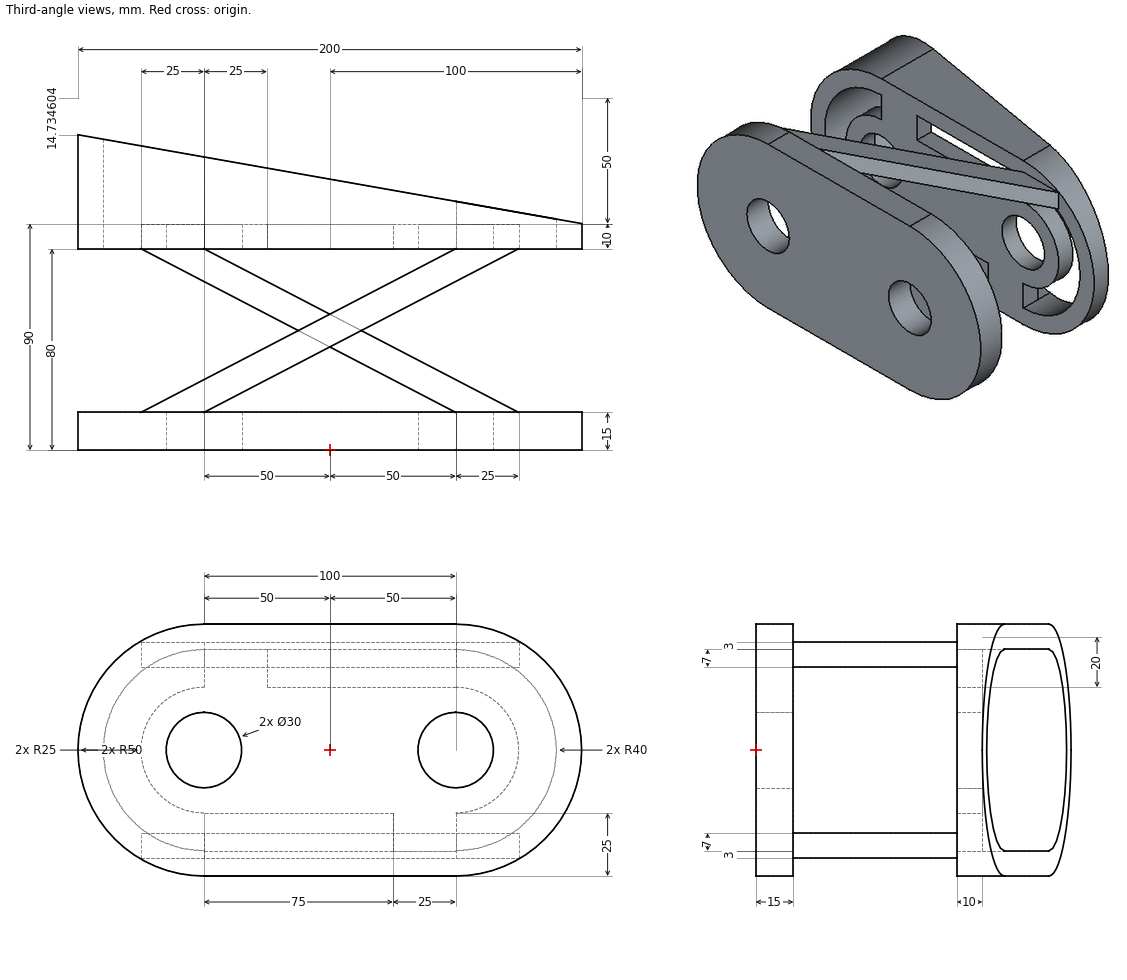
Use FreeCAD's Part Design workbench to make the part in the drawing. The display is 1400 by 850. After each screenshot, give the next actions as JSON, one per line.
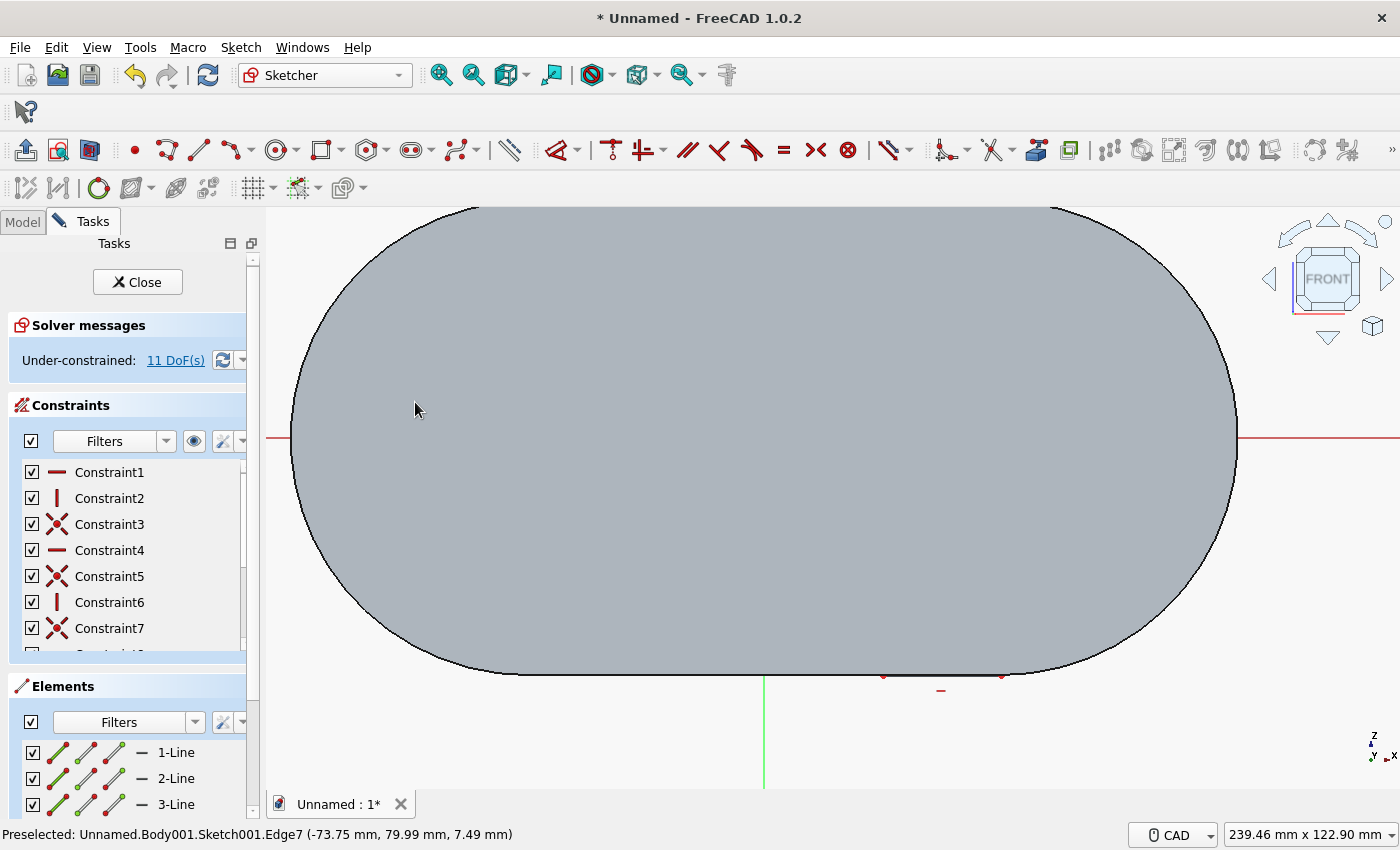
{"action": "left_click", "coordinate": [670, 321]}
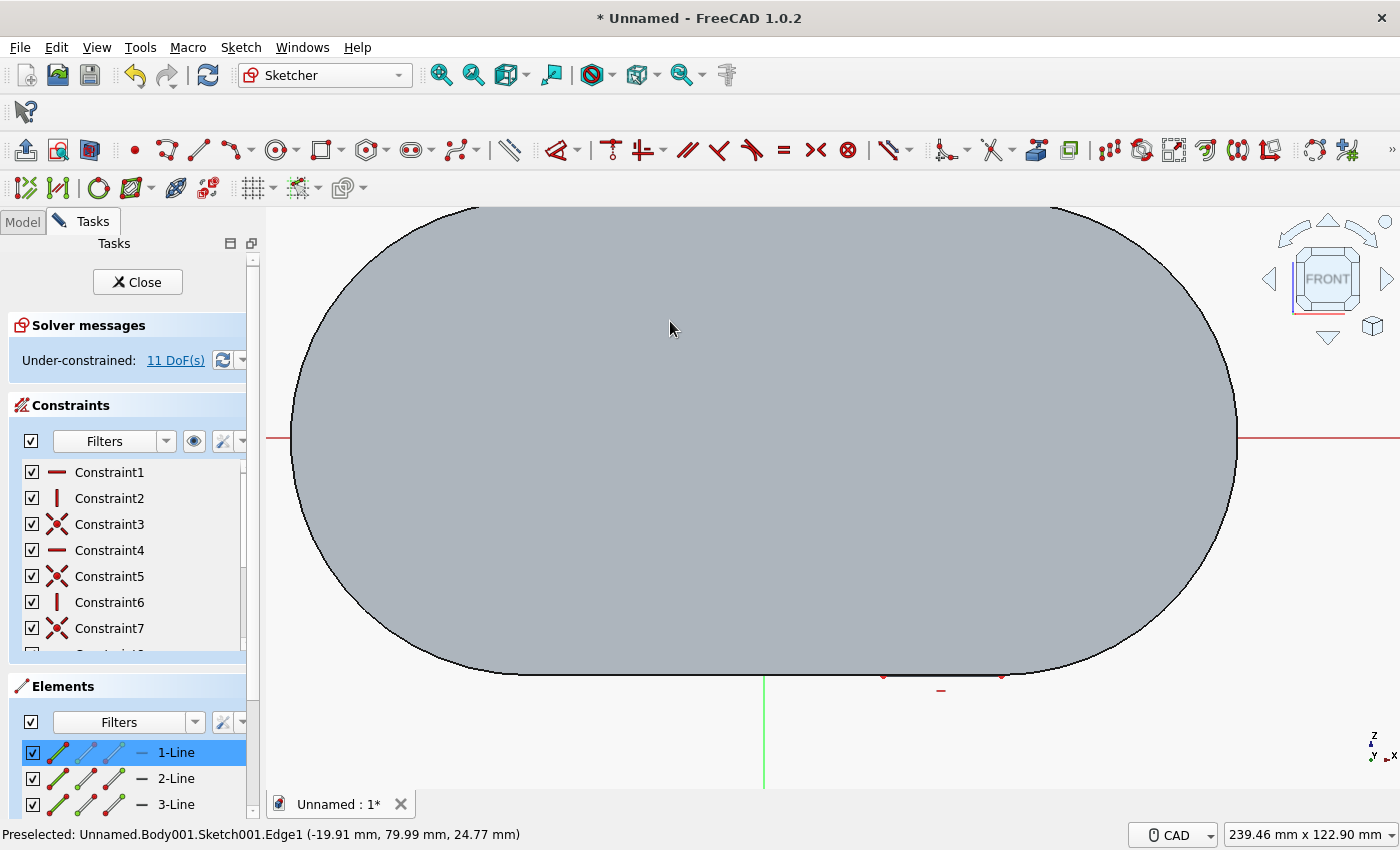
{"action": "left_click", "coordinate": [1097, 509]}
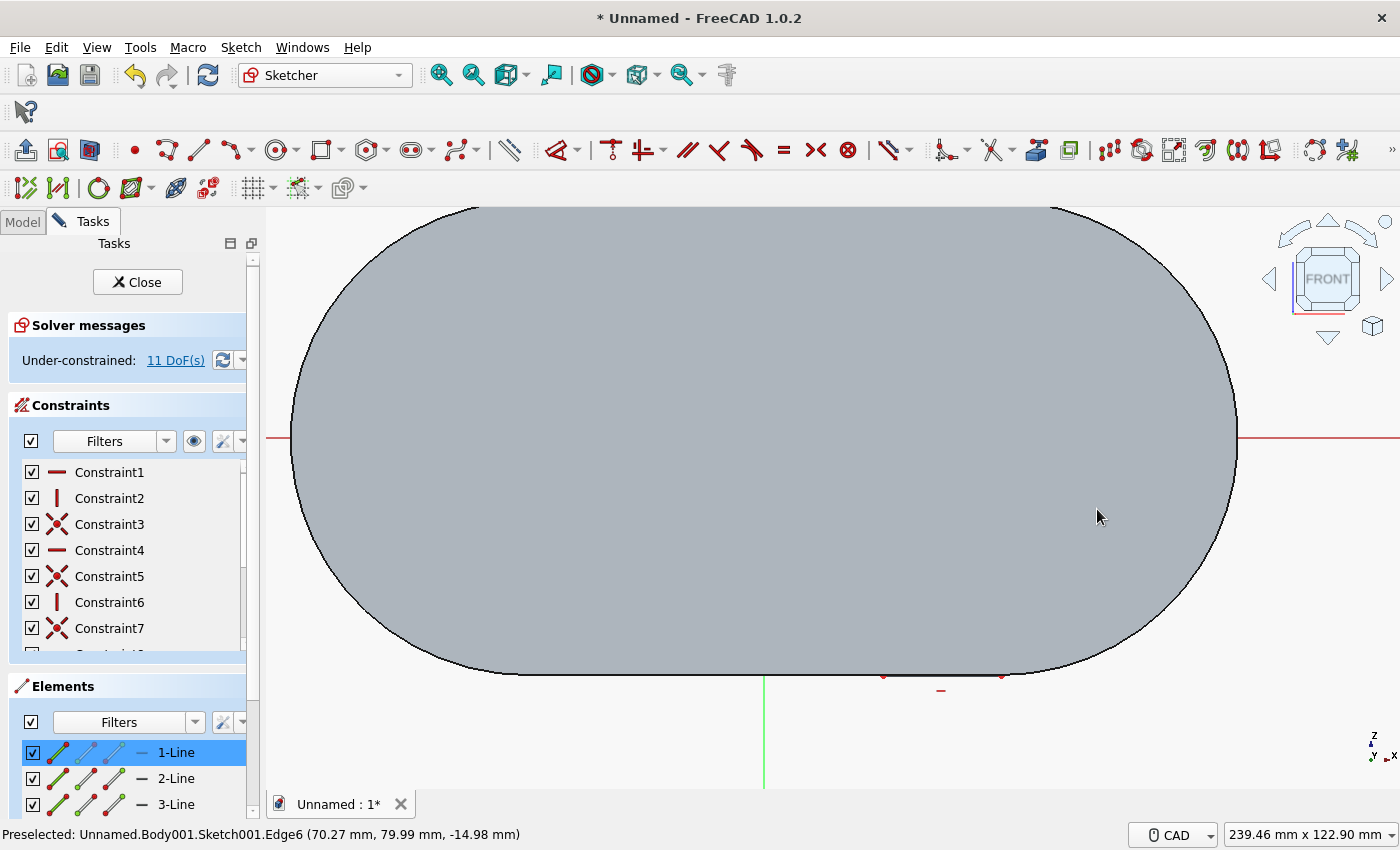
{"action": "left_click", "coordinate": [752, 150]}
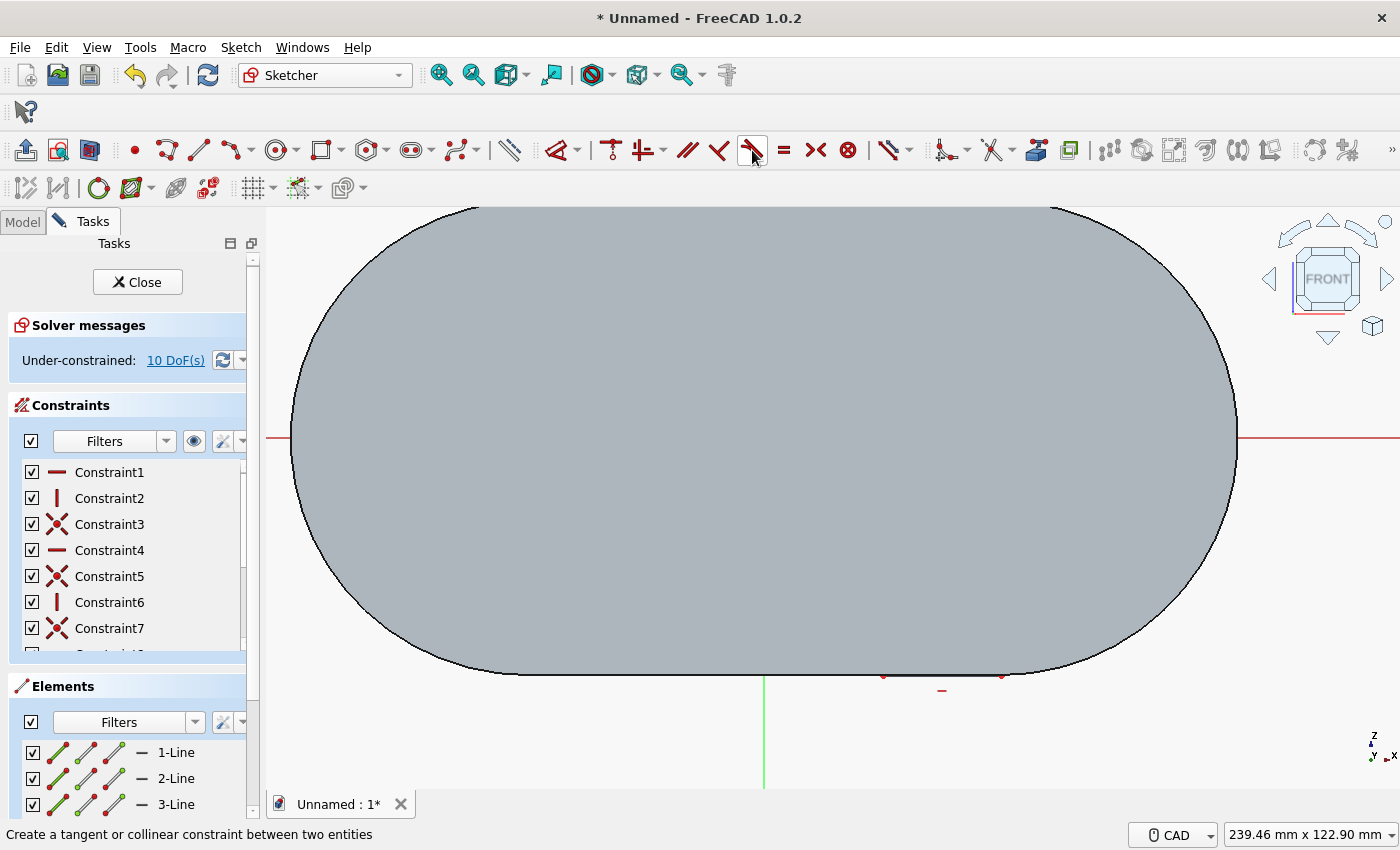
{"action": "left_click", "coordinate": [670, 321]}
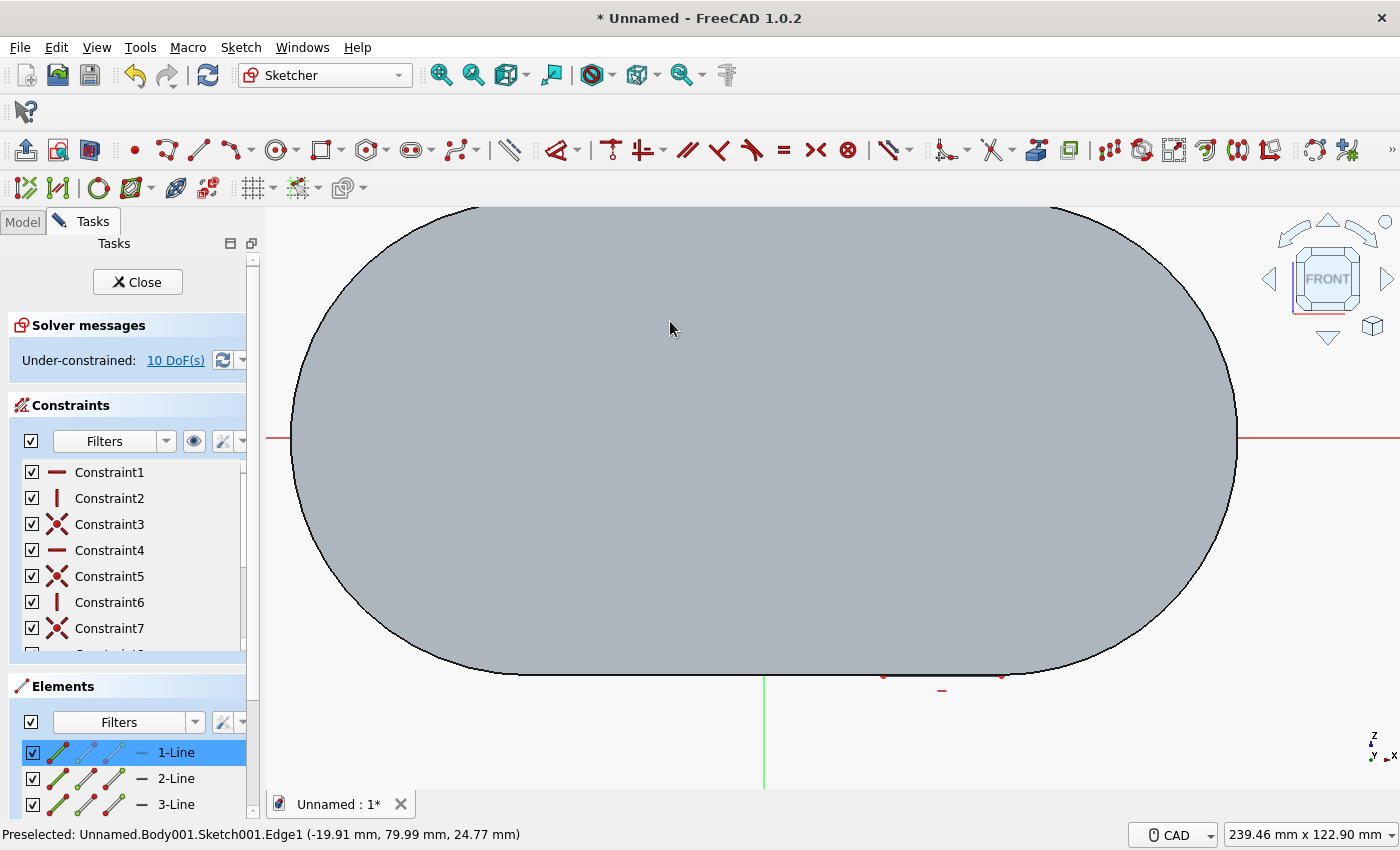
{"action": "left_click", "coordinate": [432, 370]}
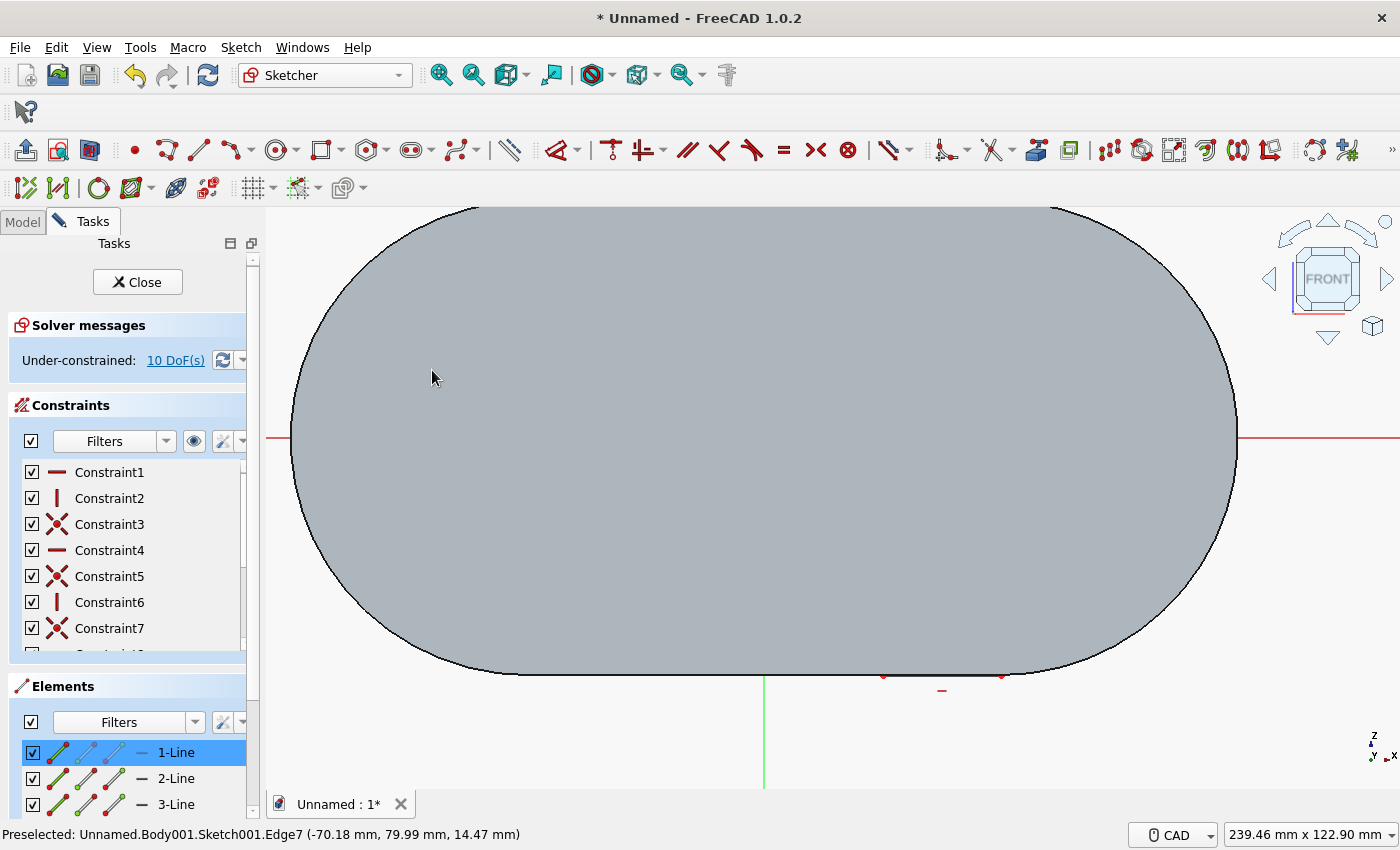
{"action": "left_click", "coordinate": [752, 150]}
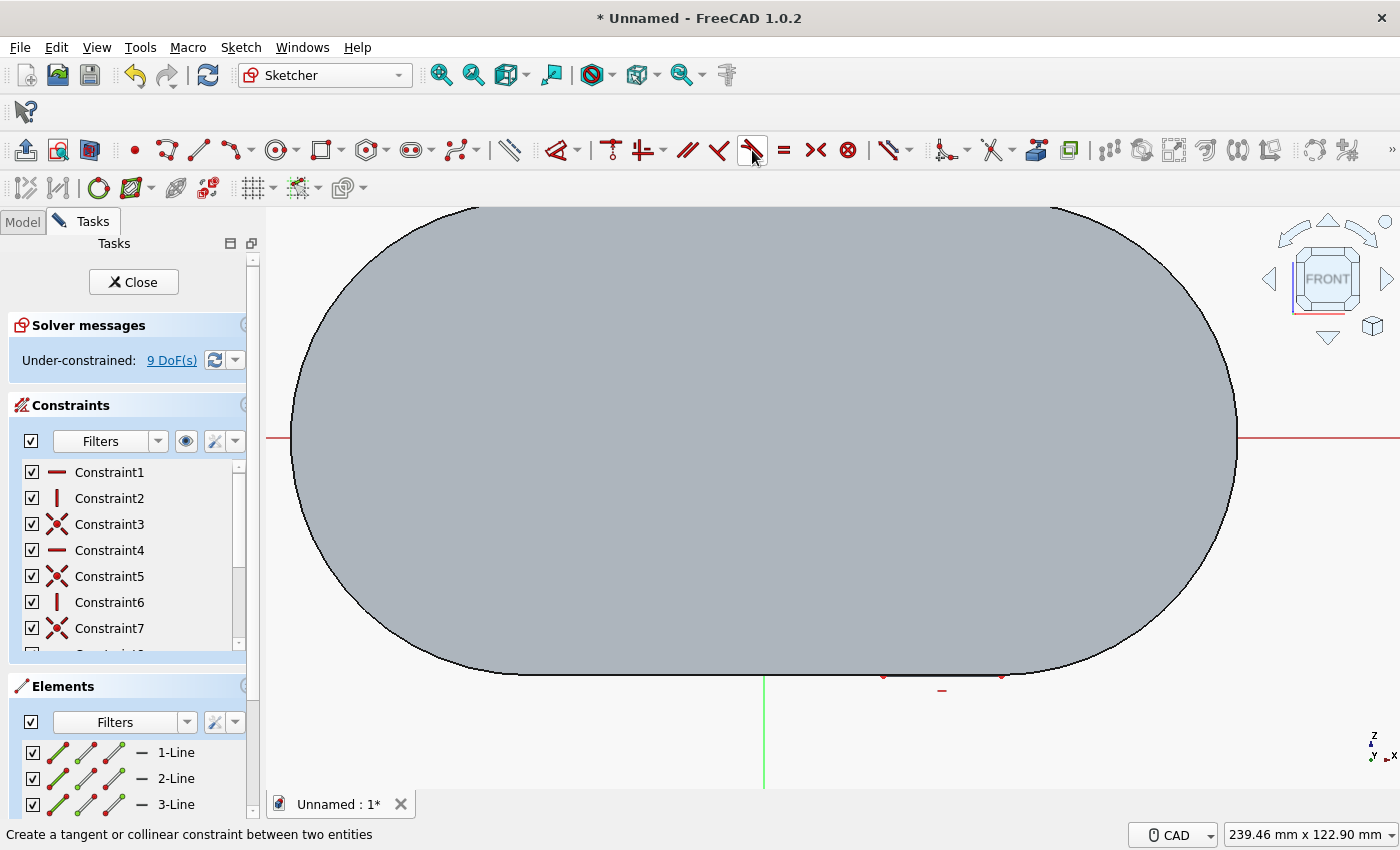
{"action": "left_click", "coordinate": [776, 558]}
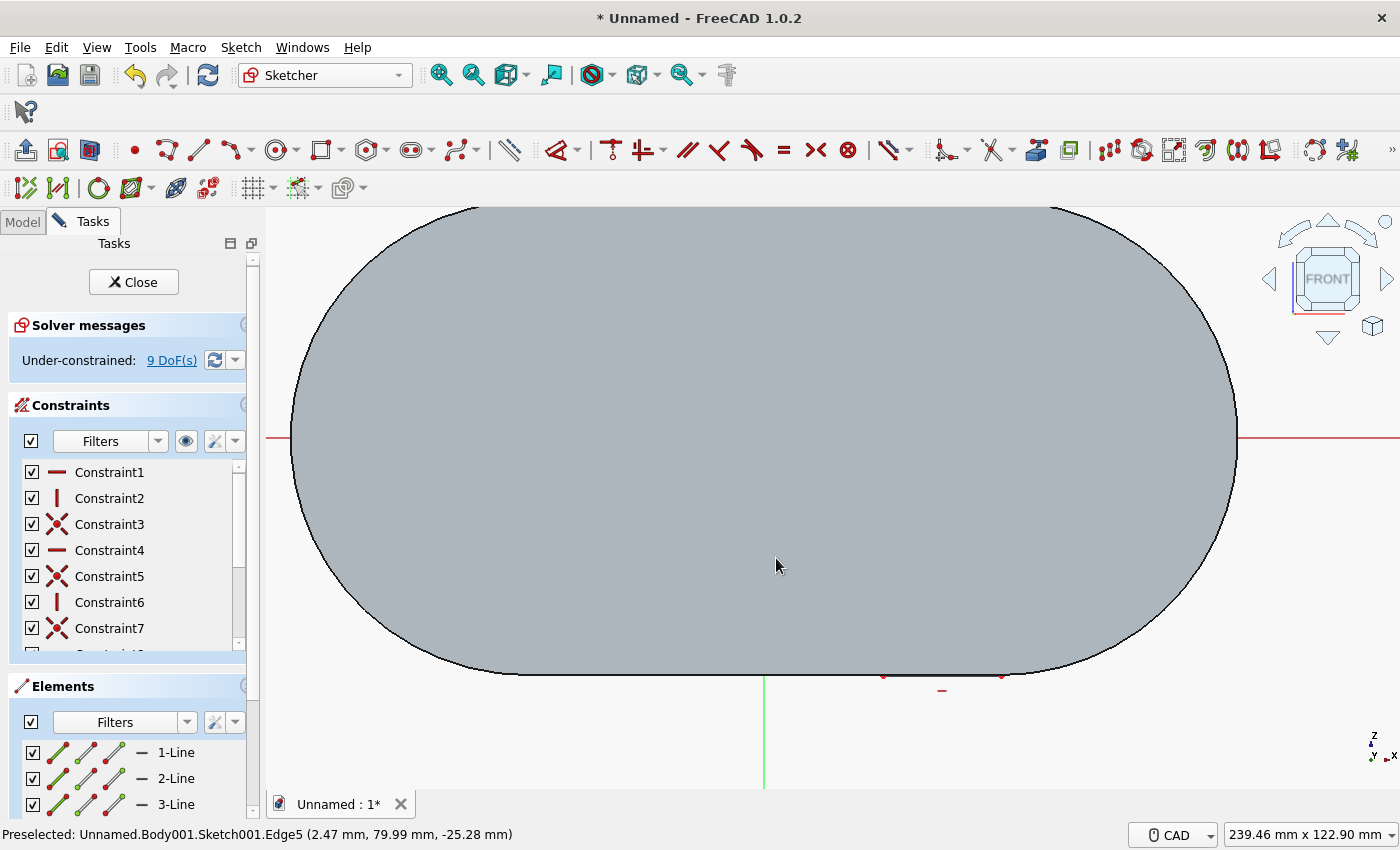
{"action": "left_click", "coordinate": [432, 370]}